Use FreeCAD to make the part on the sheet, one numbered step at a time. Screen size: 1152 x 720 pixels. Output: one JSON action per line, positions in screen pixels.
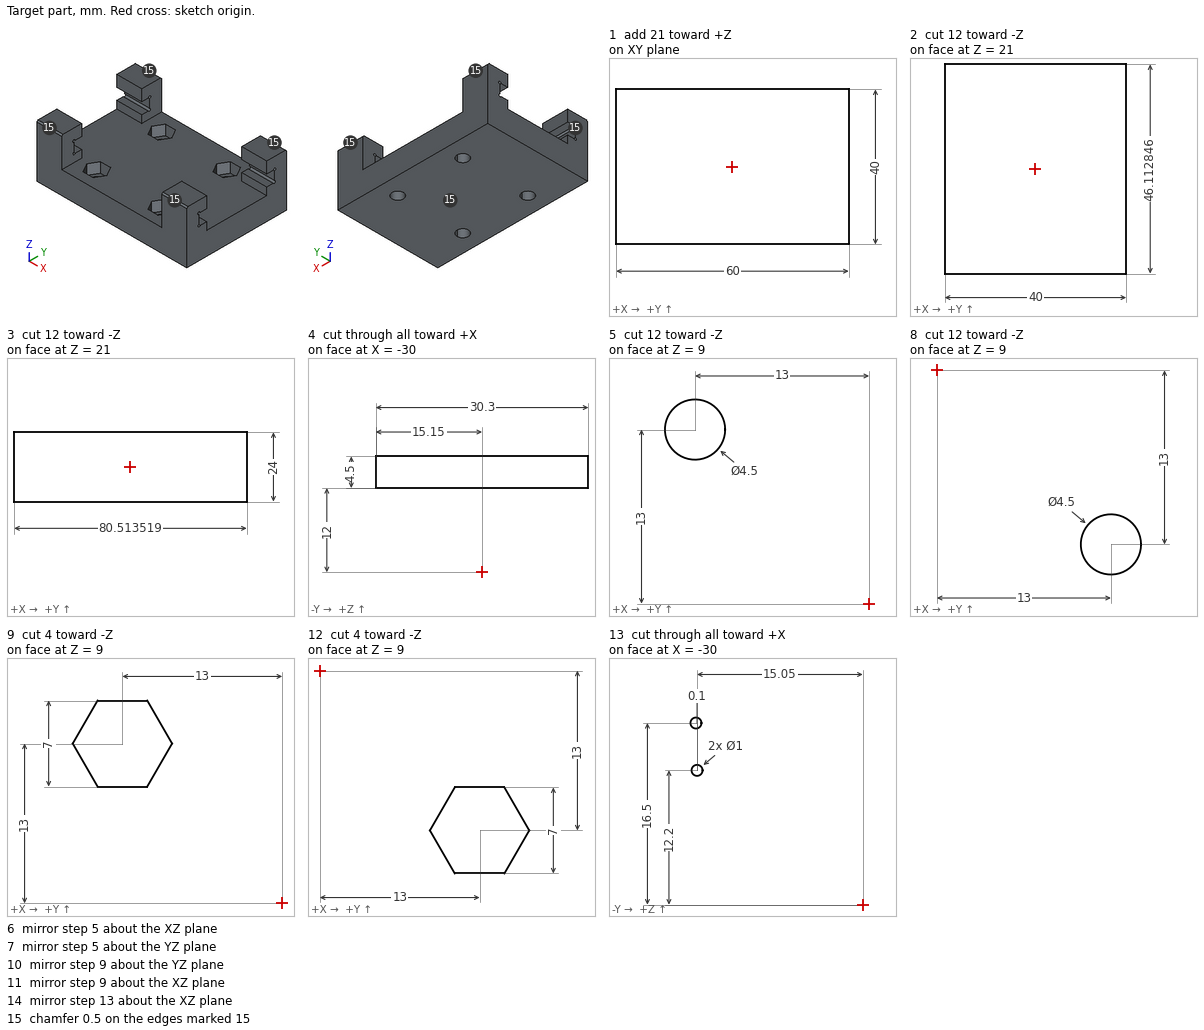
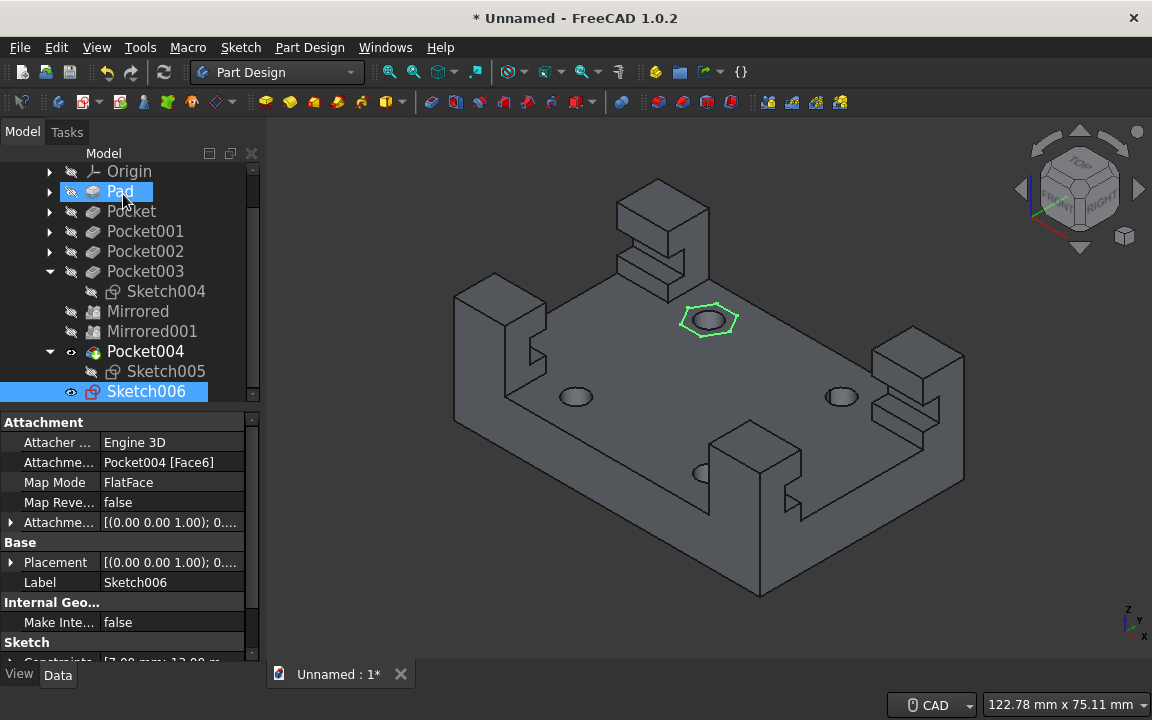
{"action": "left_click", "coordinate": [432, 102]}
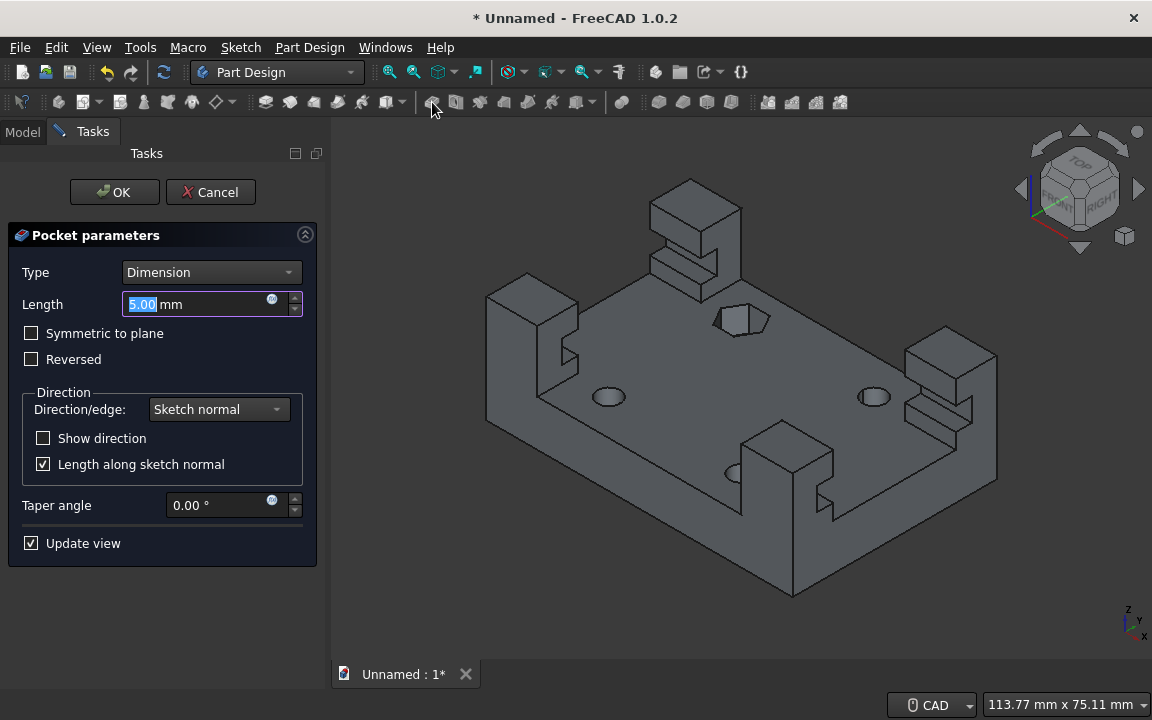
{"action": "type", "text": "4"}
{"action": "key", "text": "Tab"}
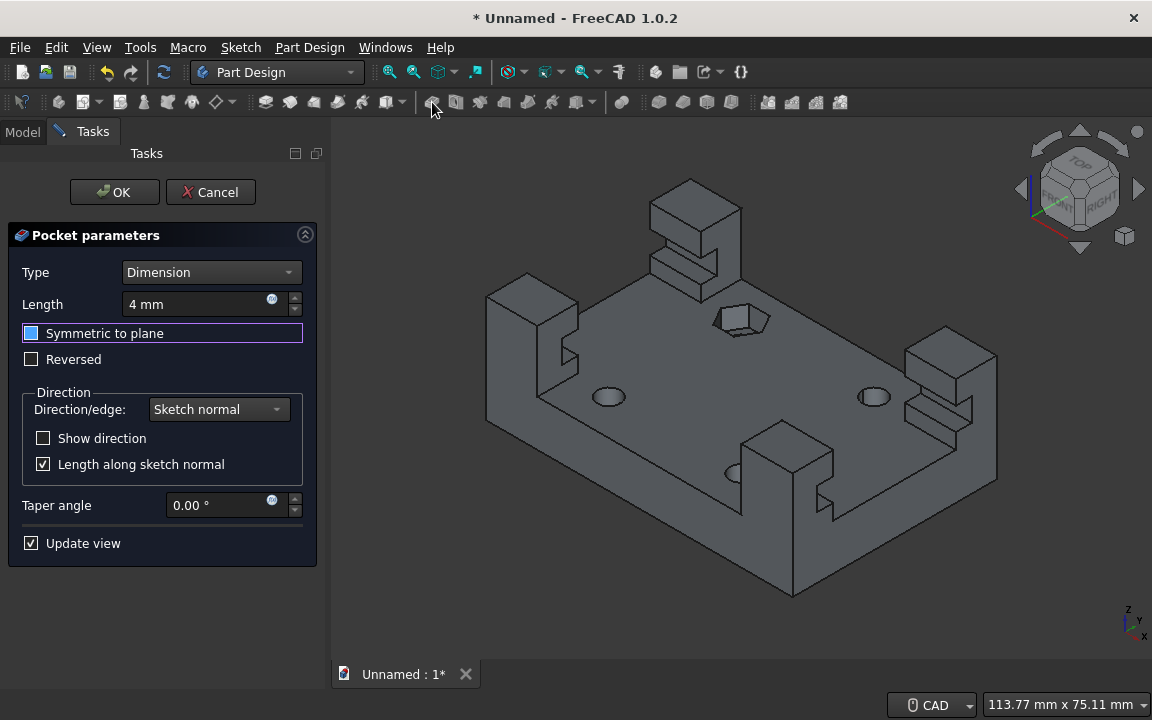
{"action": "left_click", "coordinate": [115, 192]}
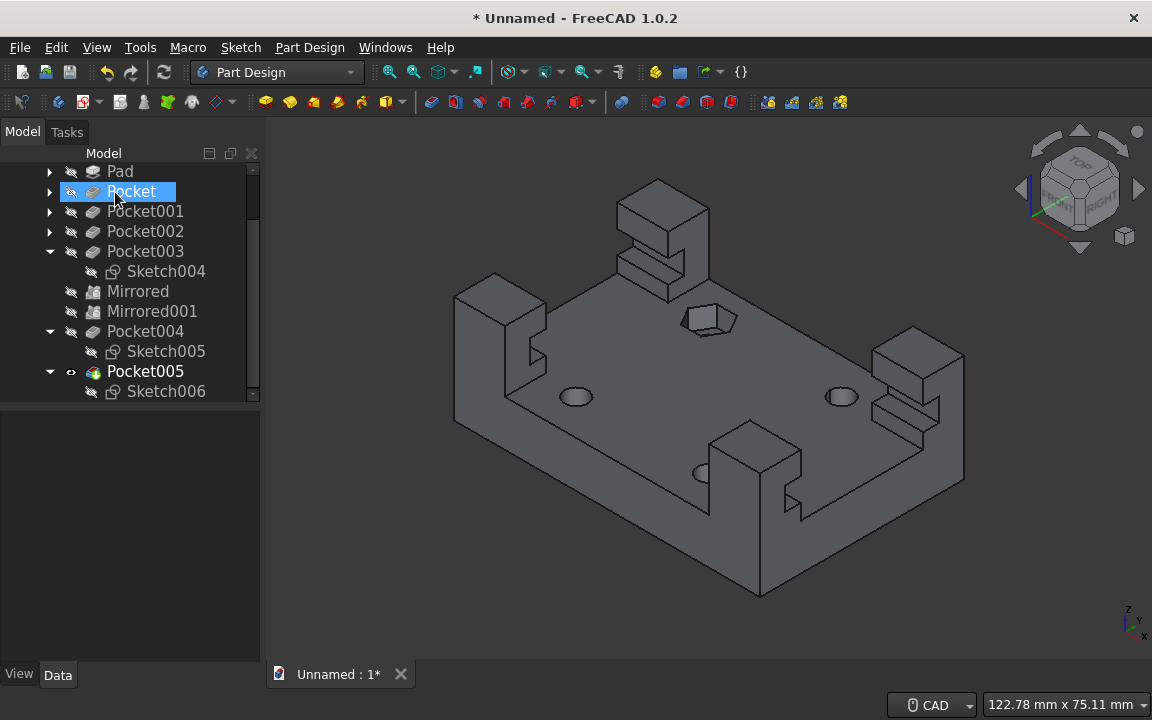
{"action": "left_click", "coordinate": [116, 372]}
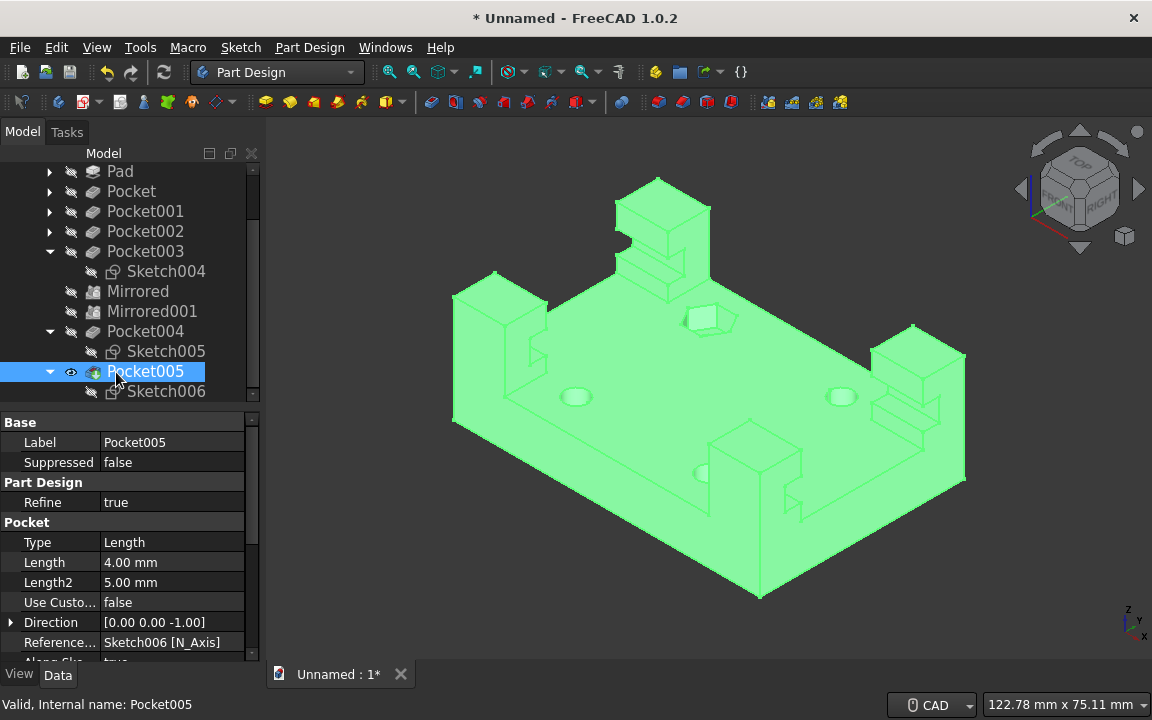
{"action": "left_click", "coordinate": [768, 102]}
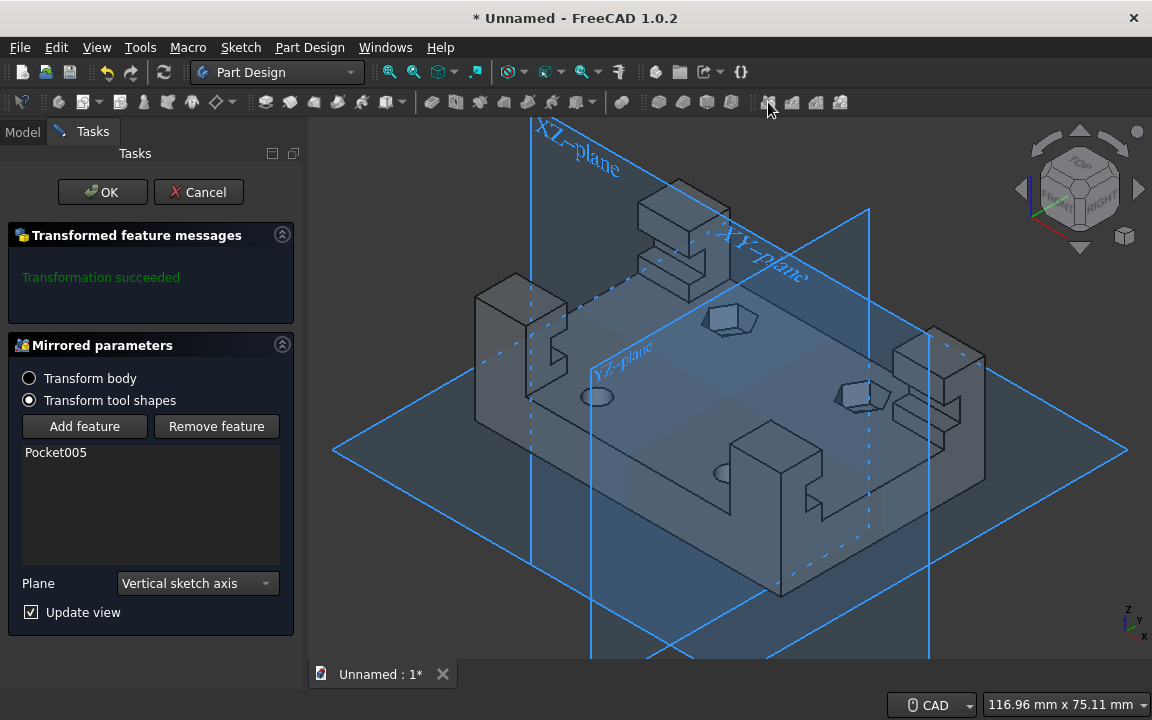
{"action": "left_click", "coordinate": [198, 584]}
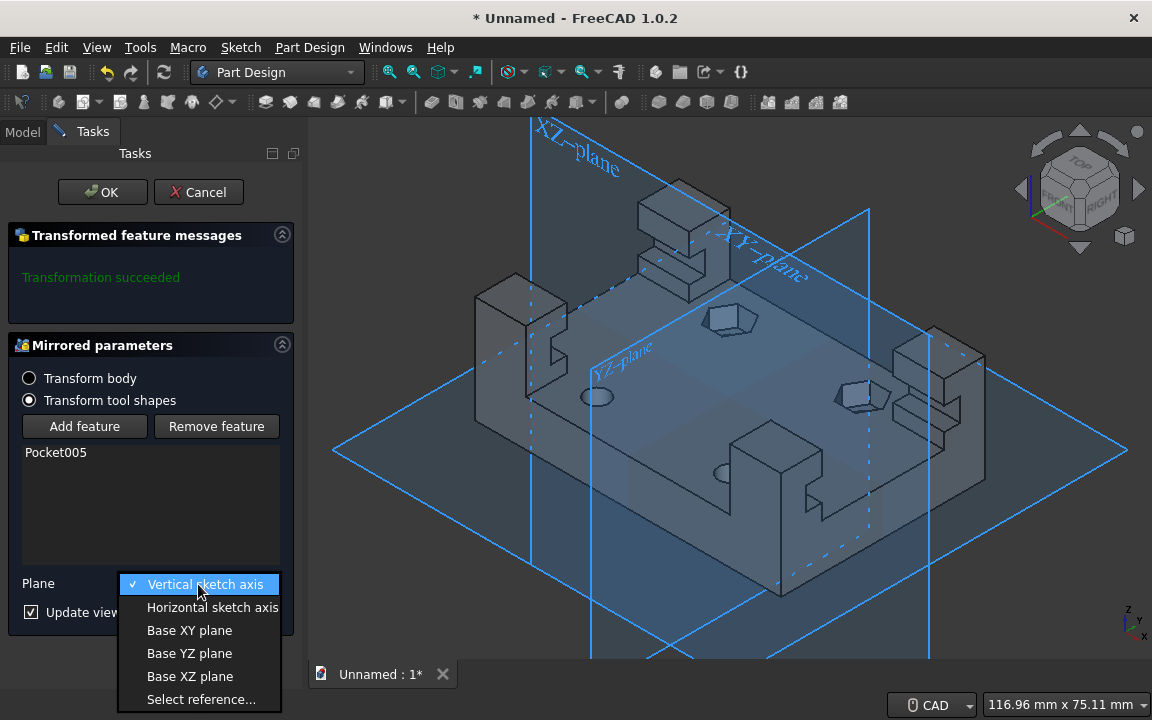
{"action": "left_click", "coordinate": [198, 654]}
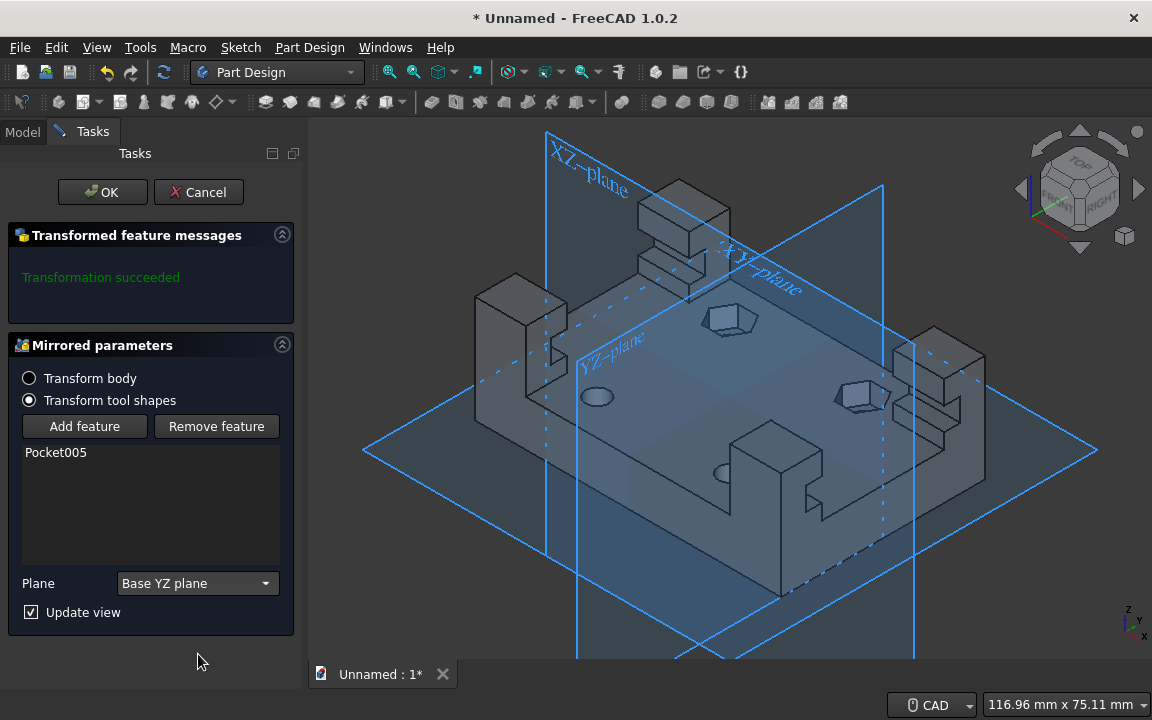
{"action": "left_click", "coordinate": [103, 192]}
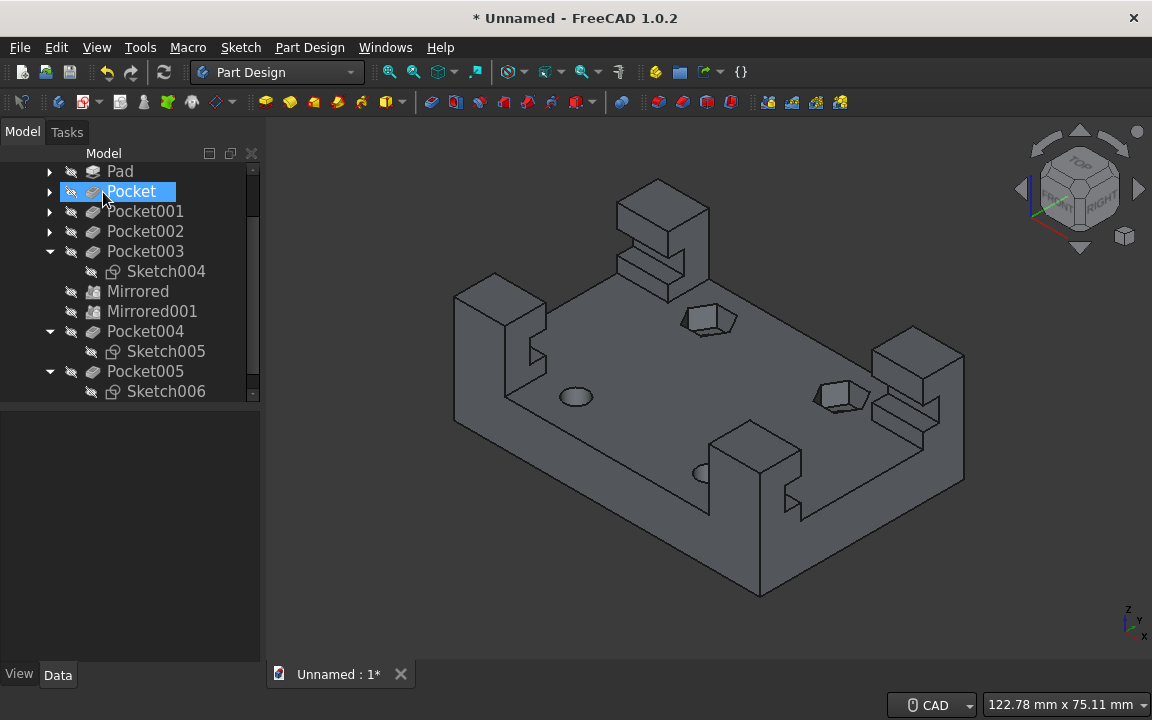
{"action": "left_click", "coordinate": [116, 372]}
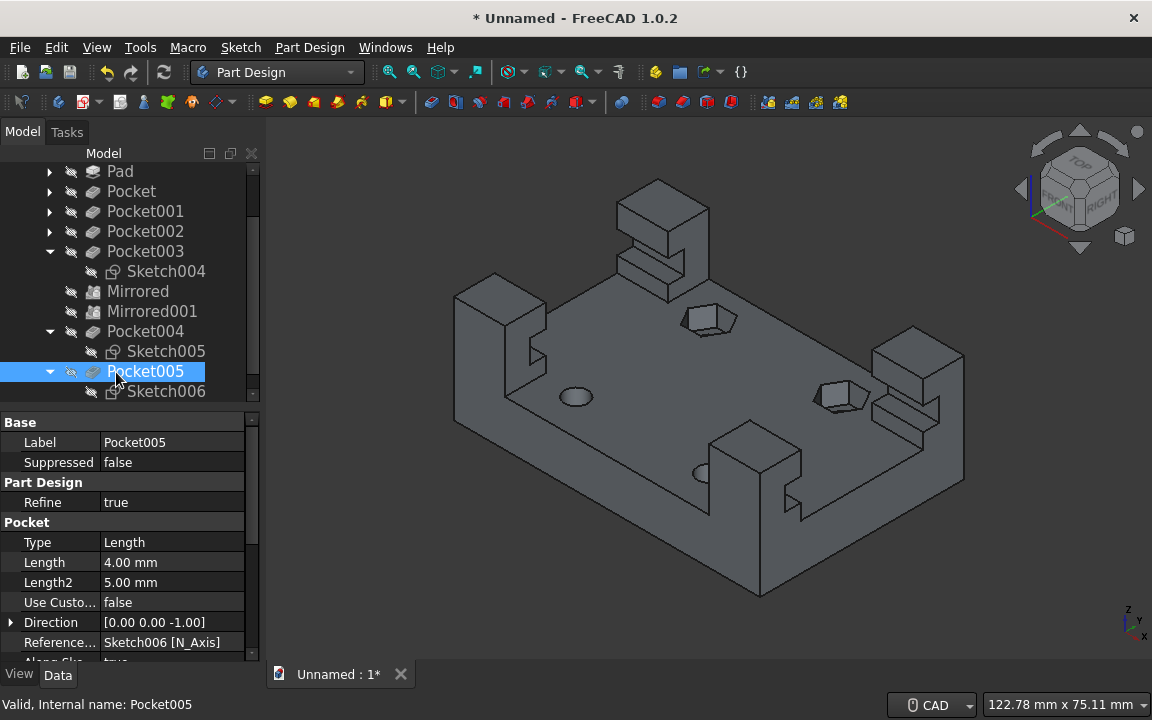
{"action": "left_click", "coordinate": [768, 102]}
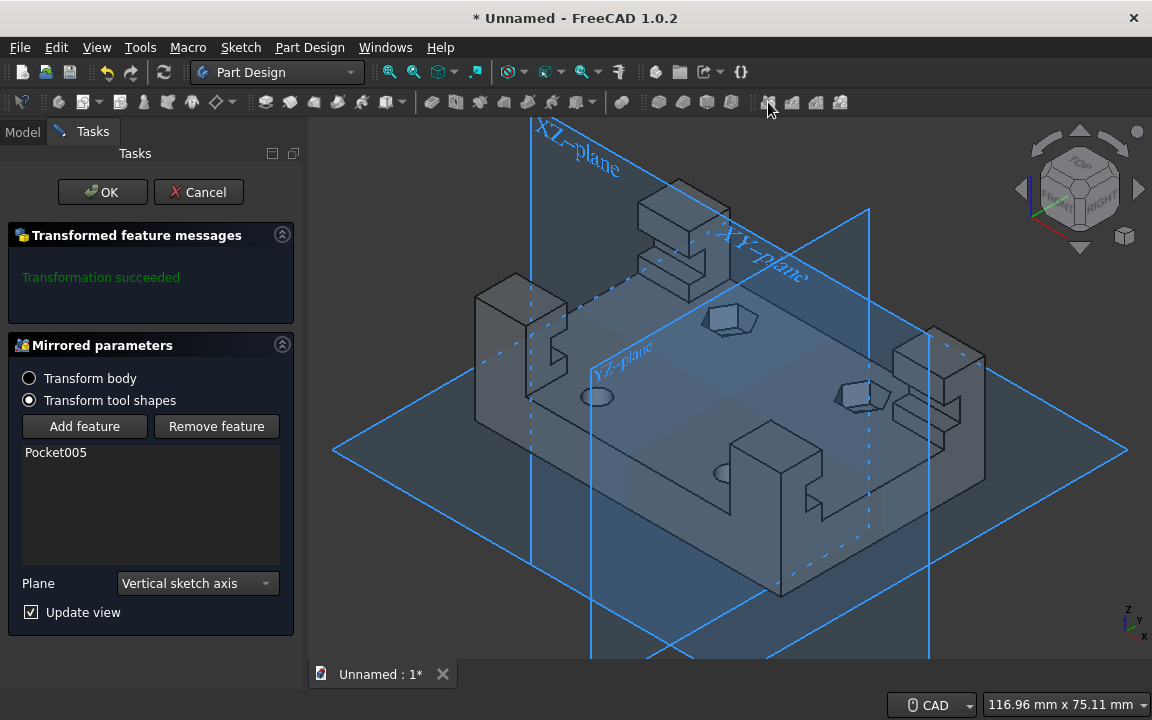
{"action": "left_click", "coordinate": [198, 584]}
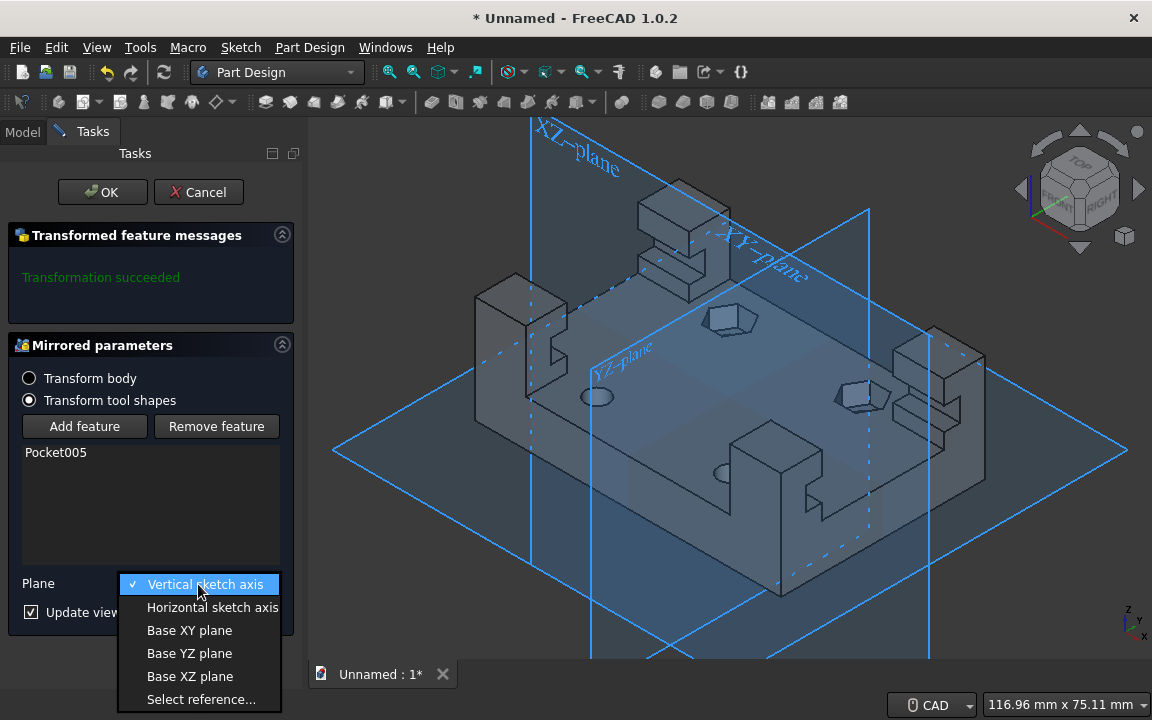
{"action": "left_click", "coordinate": [198, 676]}